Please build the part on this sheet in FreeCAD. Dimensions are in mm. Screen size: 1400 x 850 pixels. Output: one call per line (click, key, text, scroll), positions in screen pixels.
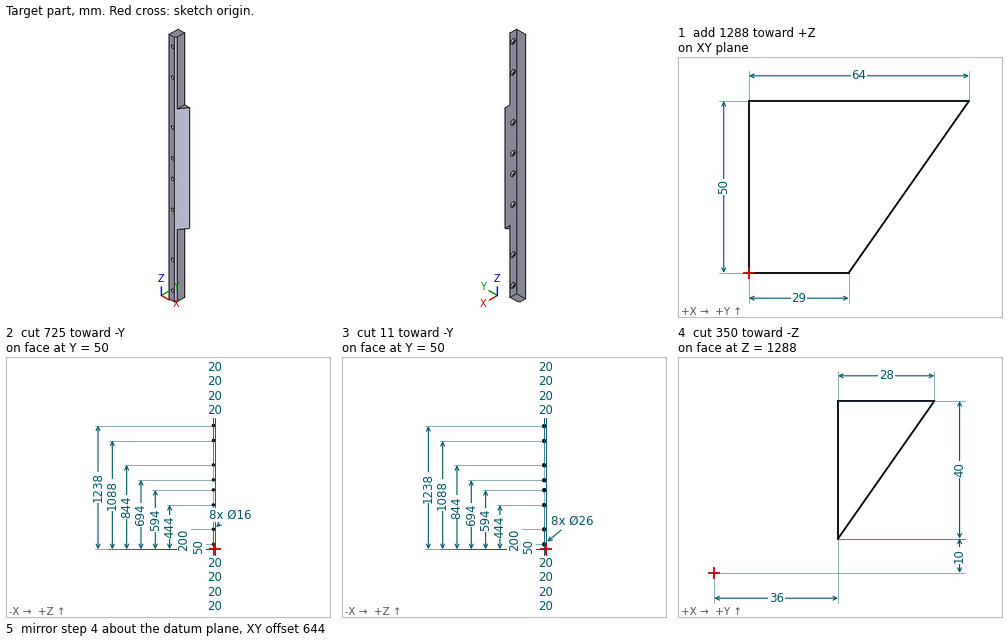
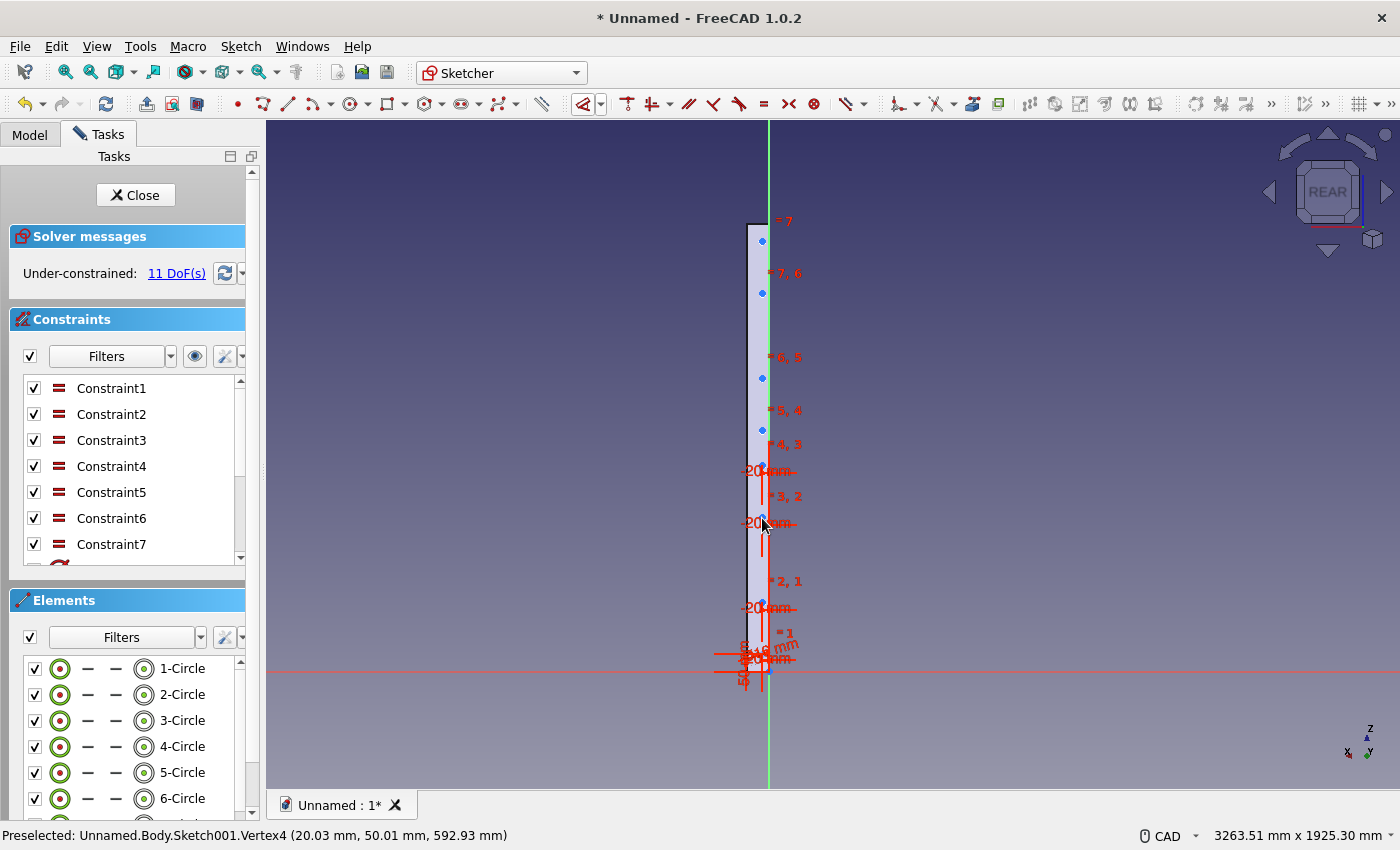
scroll(762, 431, up, 9)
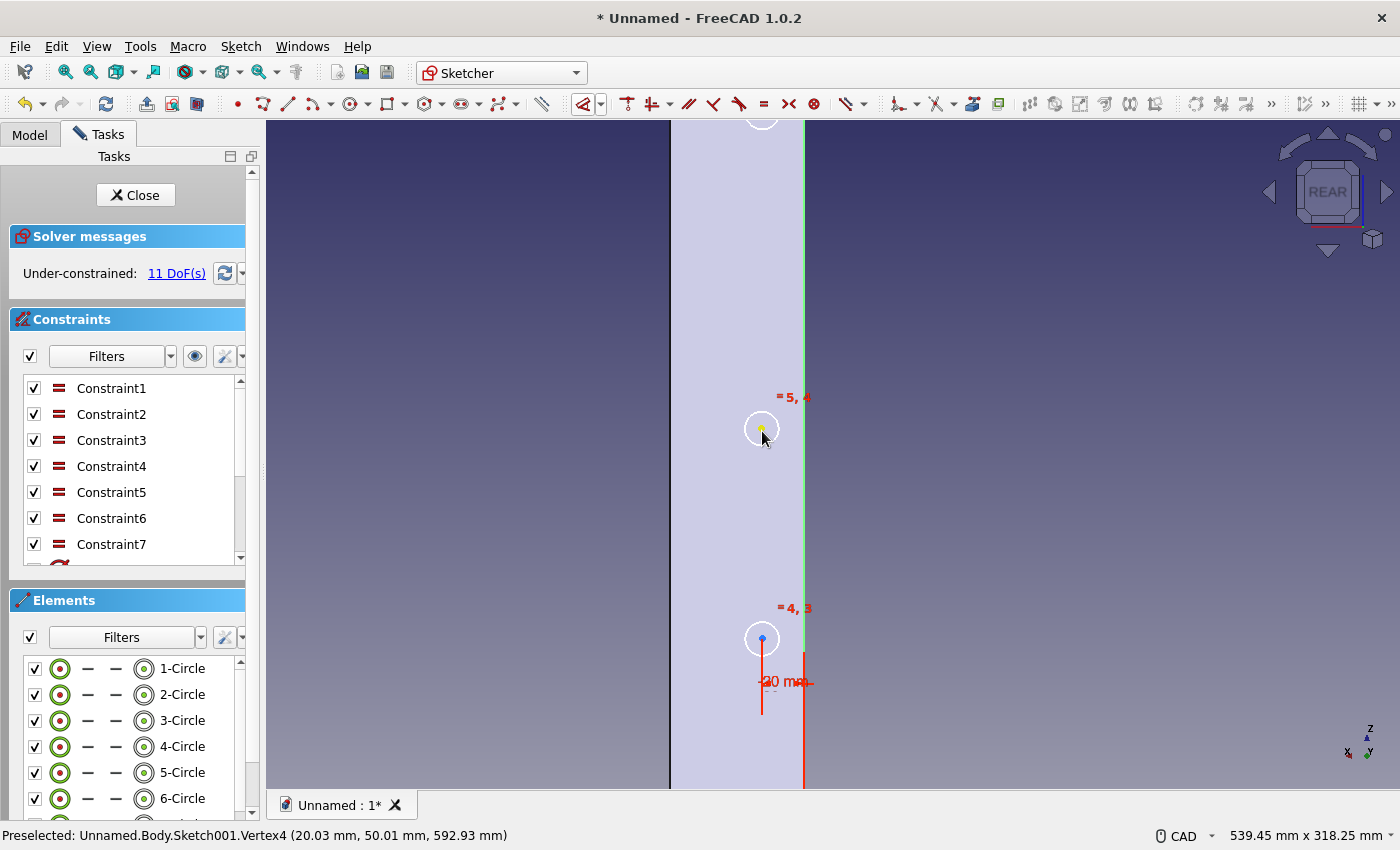
click(762, 429)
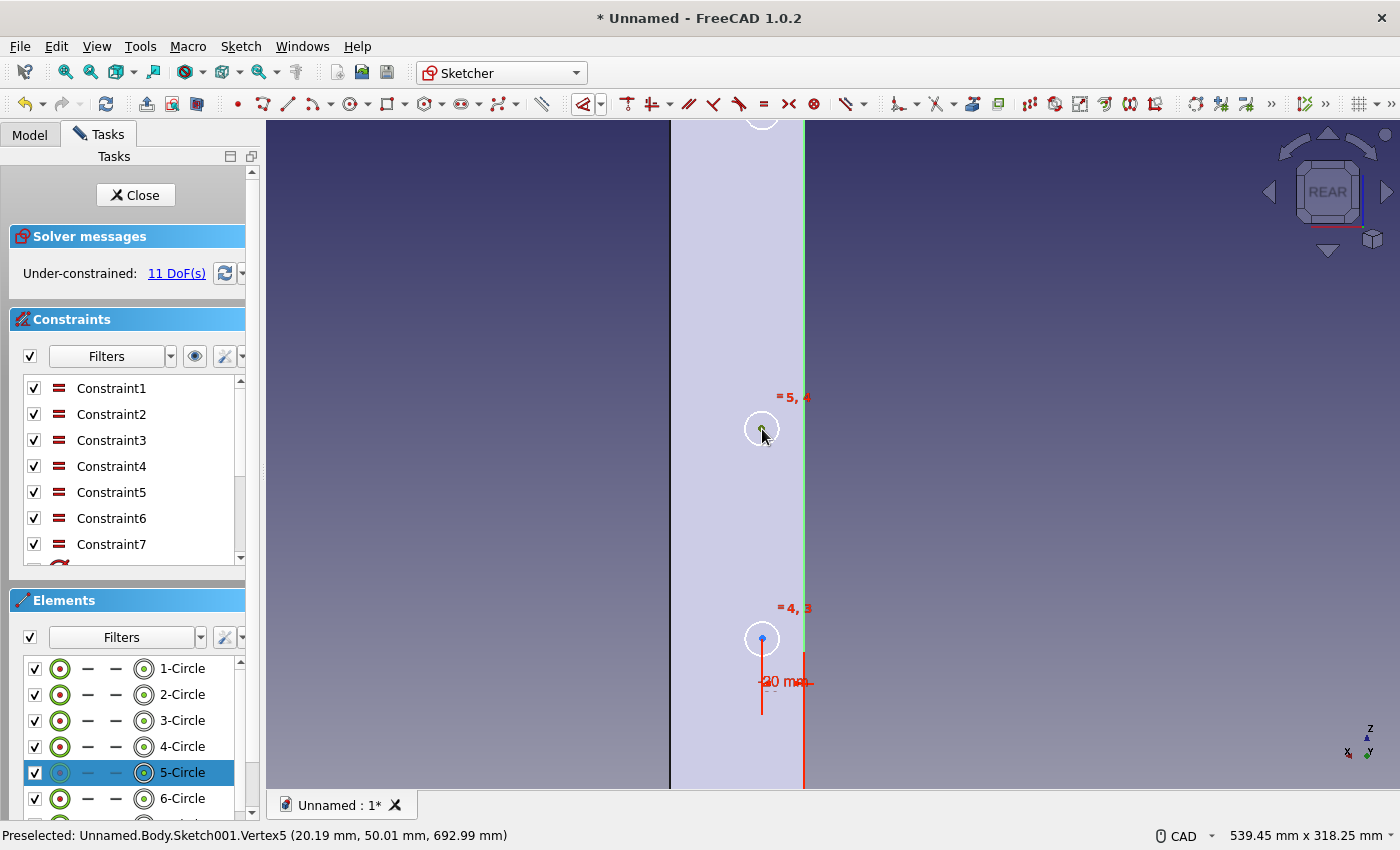
key(l)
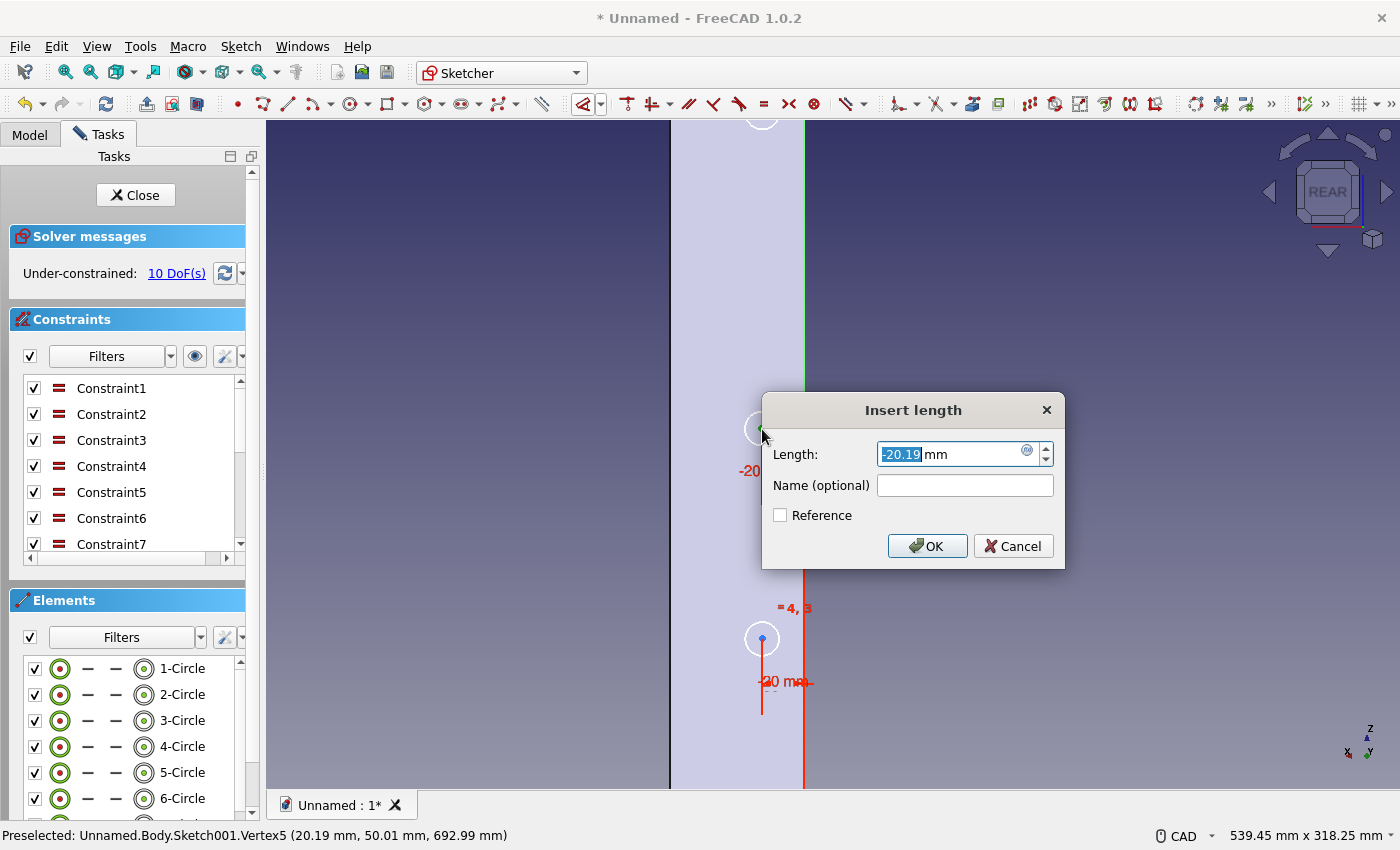
text(-20)
key(Return)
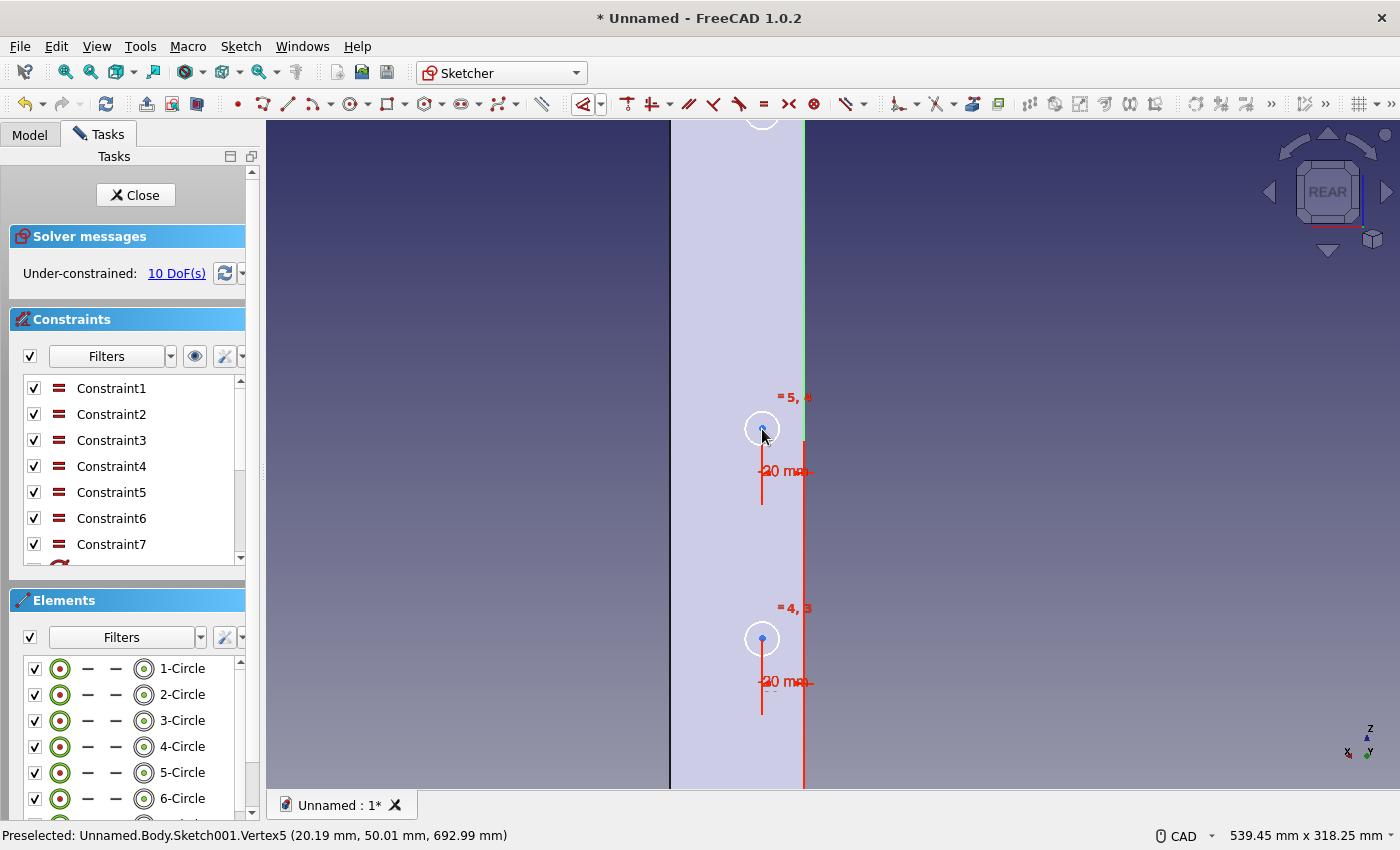
scroll(762, 430, down, 9)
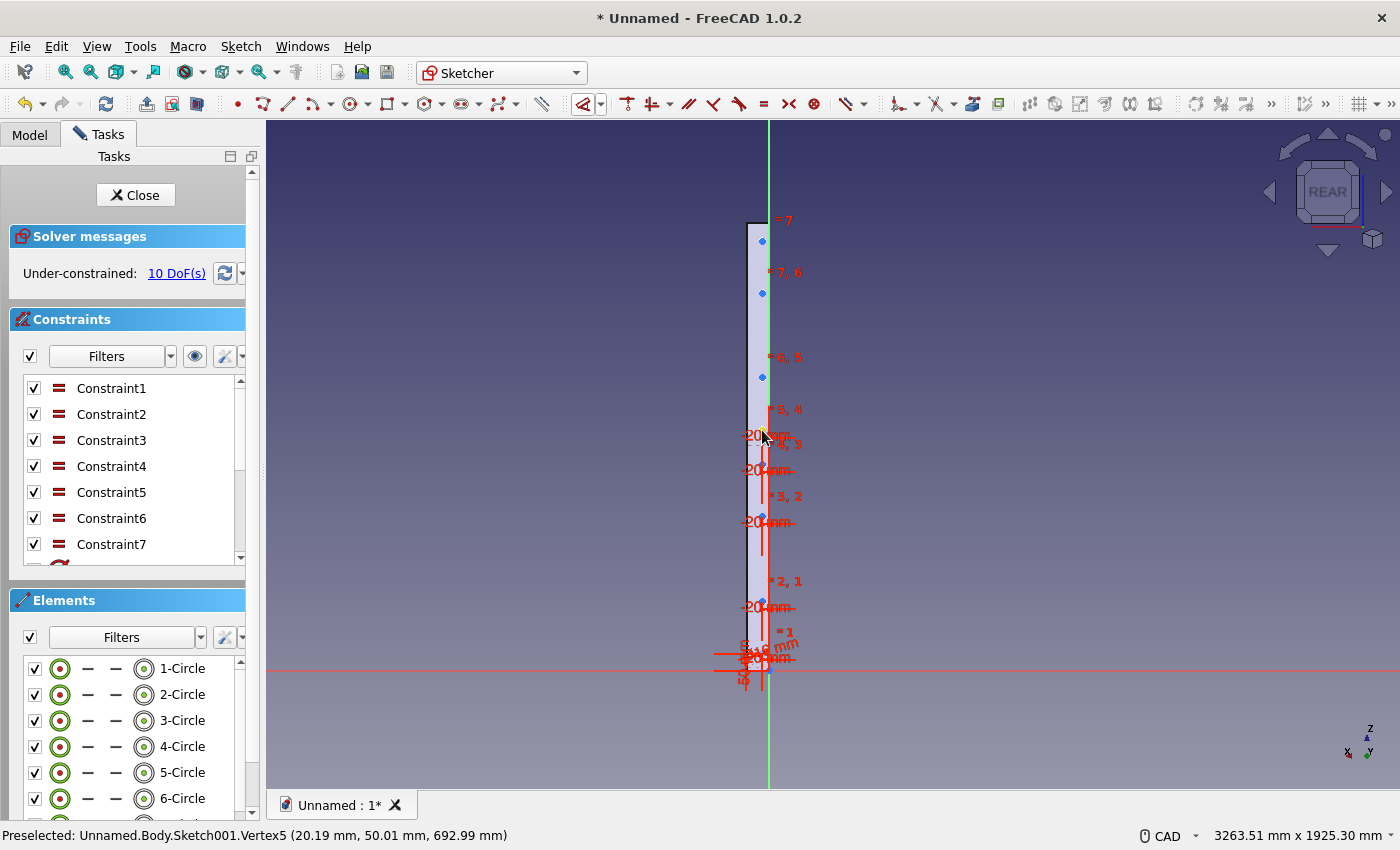
scroll(762, 378, up, 9)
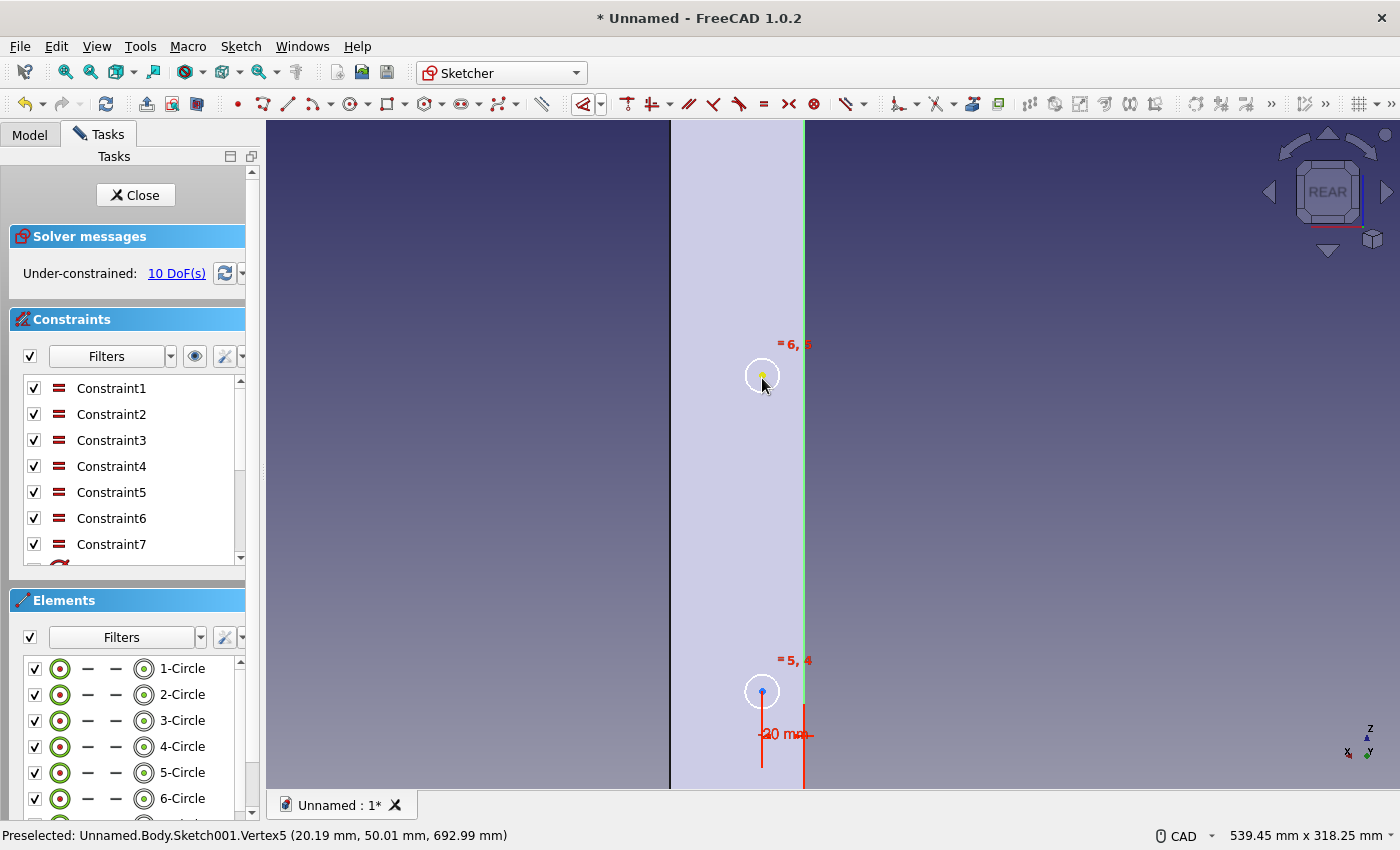
click(762, 376)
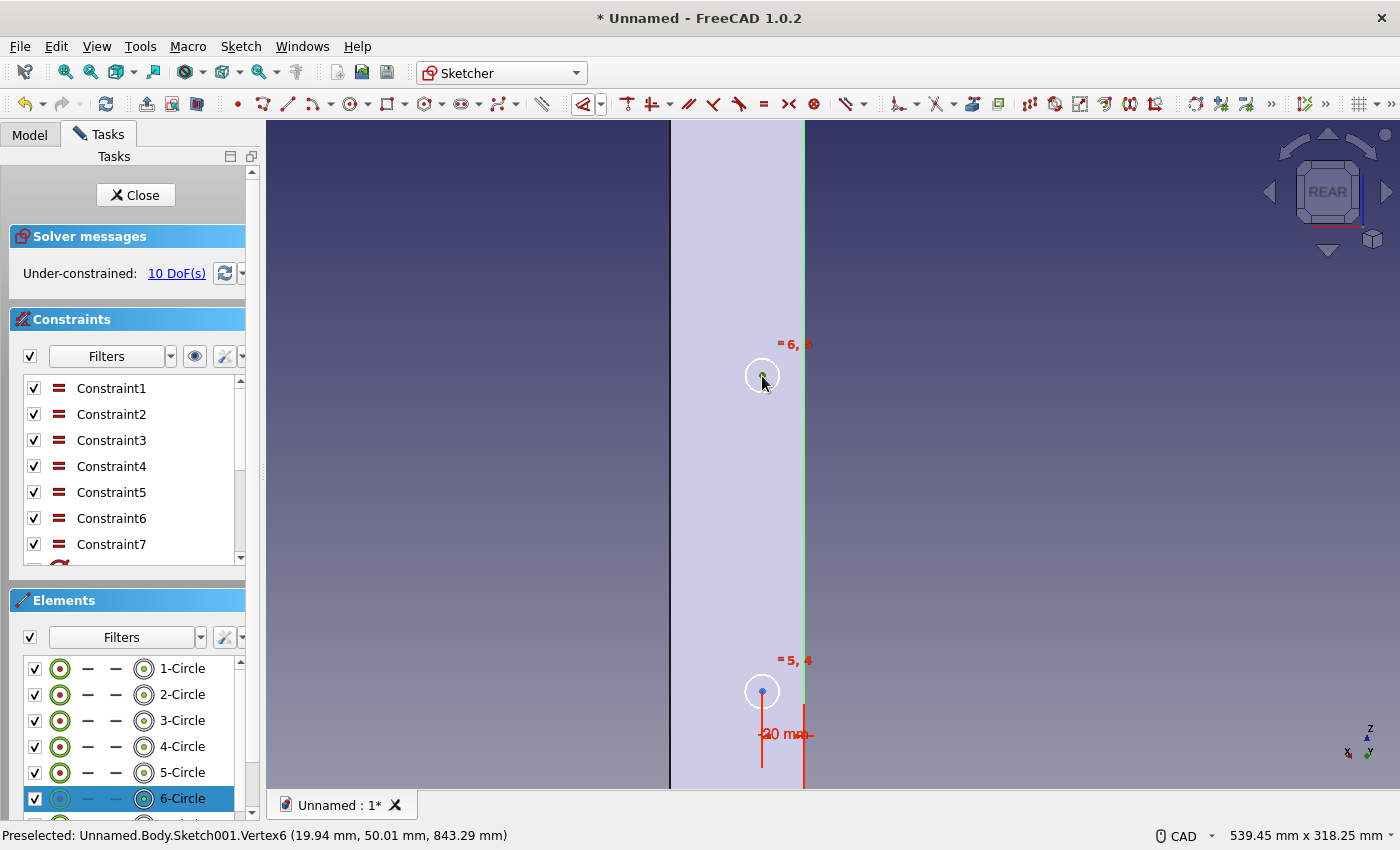
key(l)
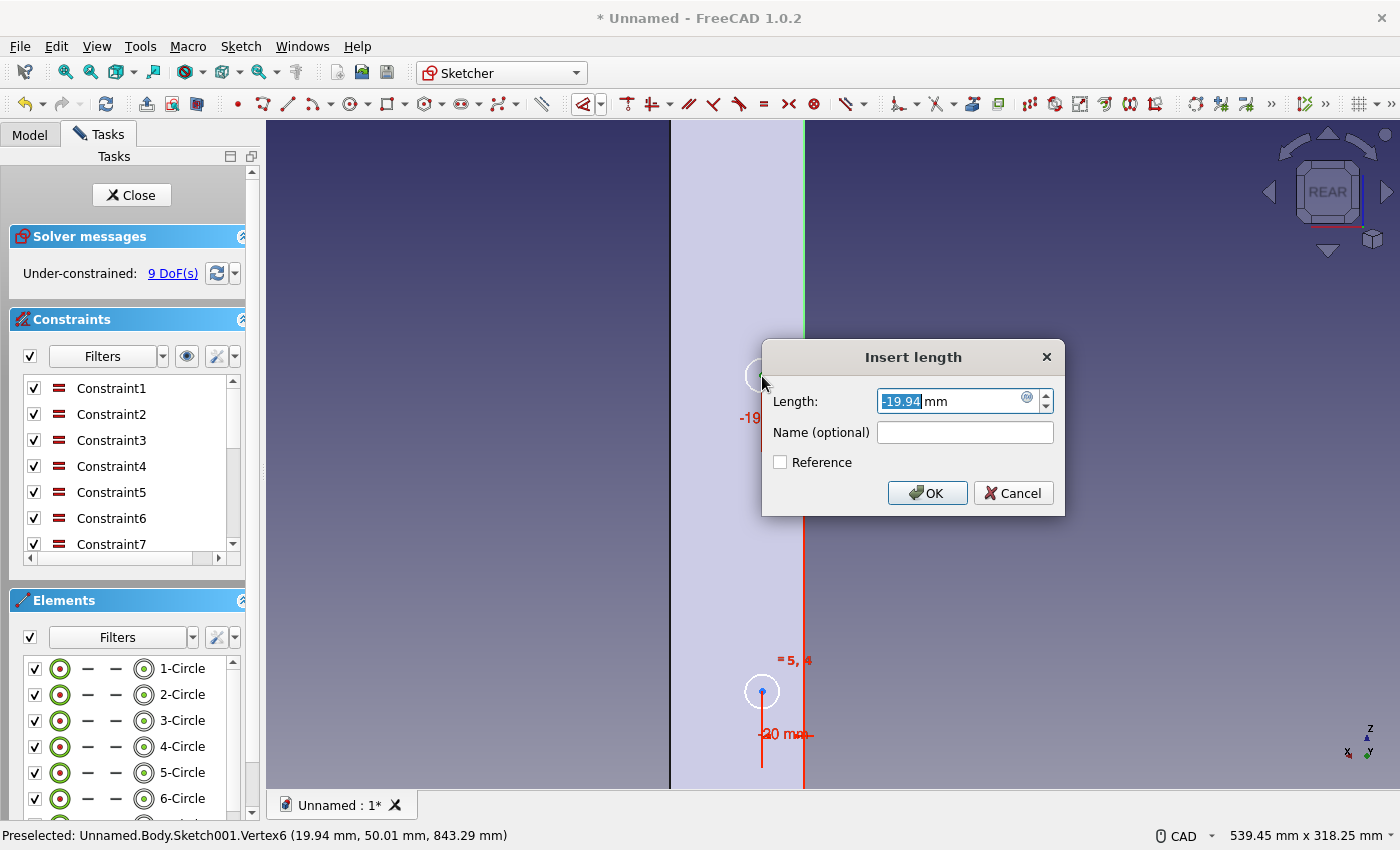
text(-20)
key(Return)